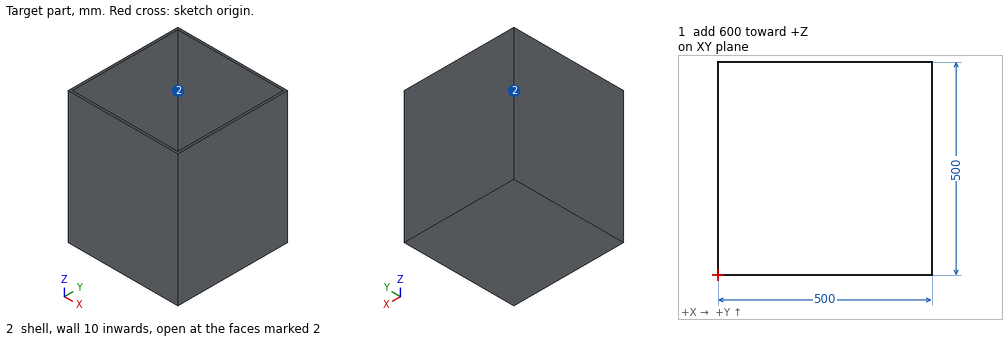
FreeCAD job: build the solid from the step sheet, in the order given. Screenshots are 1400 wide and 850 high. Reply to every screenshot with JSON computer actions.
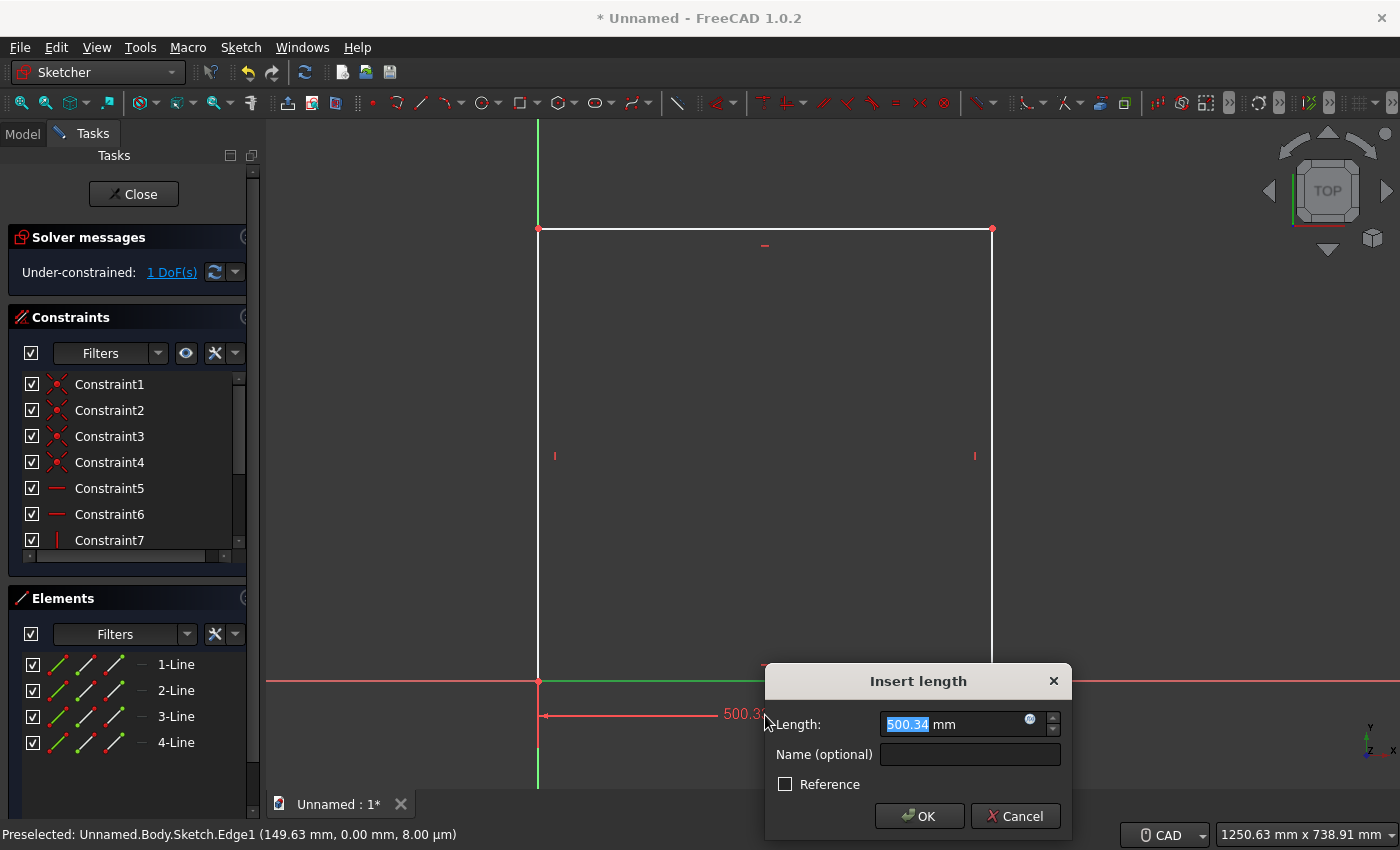
{"action": "type", "text": "500"}
{"action": "key", "text": "Return"}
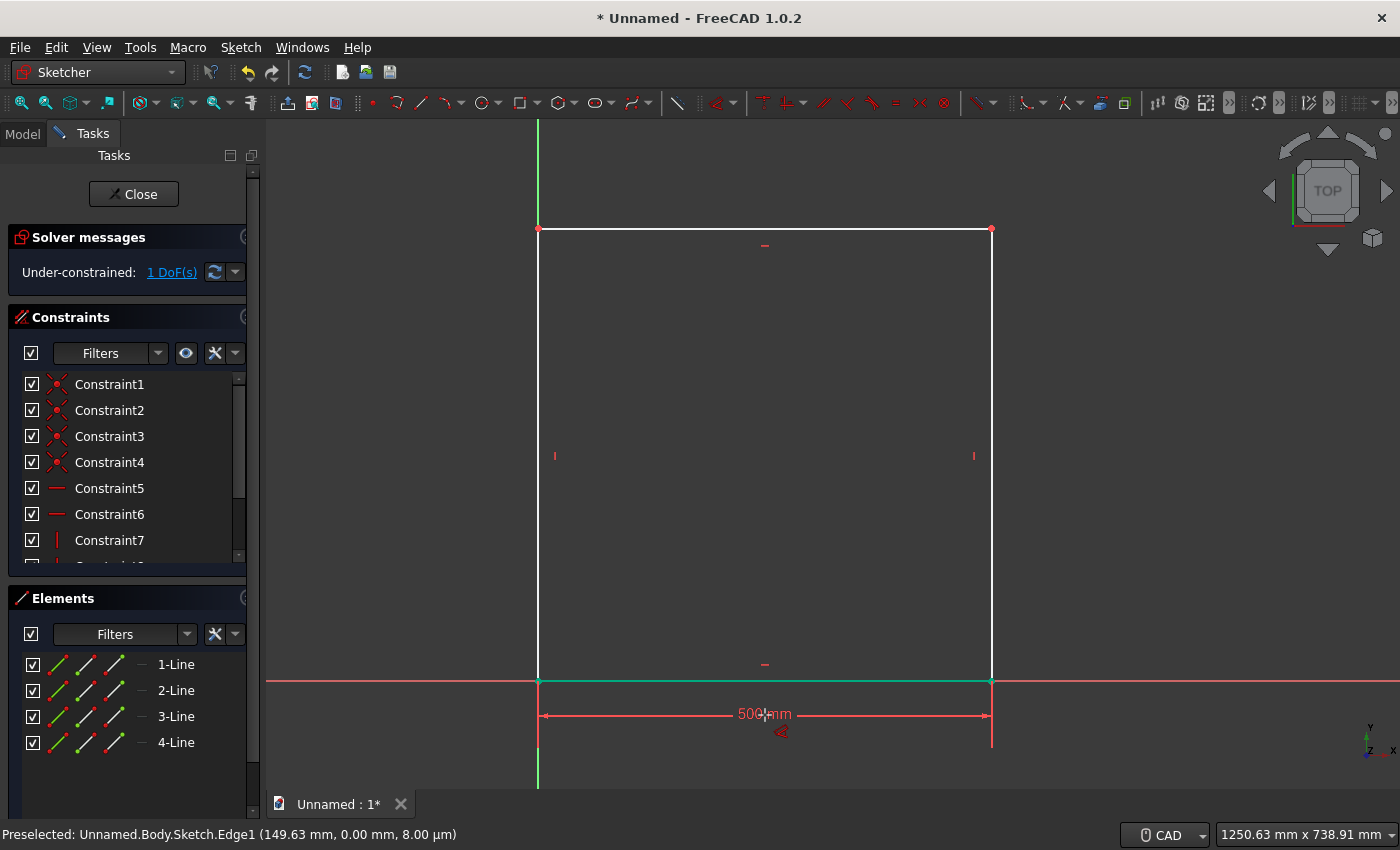
{"action": "left_click", "coordinate": [992, 546]}
{"action": "left_click", "coordinate": [1026, 455]}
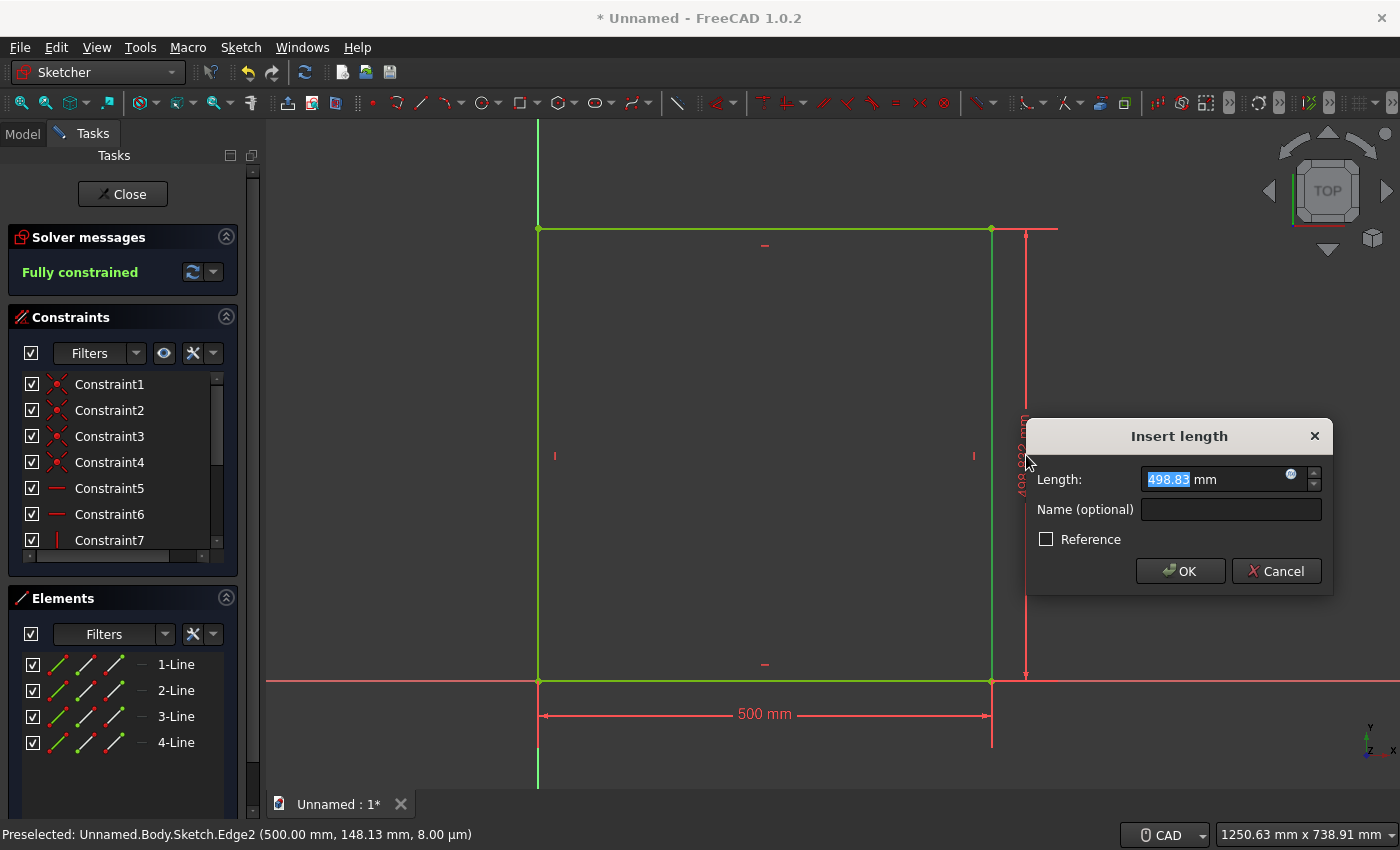
{"action": "type", "text": "500"}
{"action": "key", "text": "Return"}
{"action": "key", "text": "Escape"}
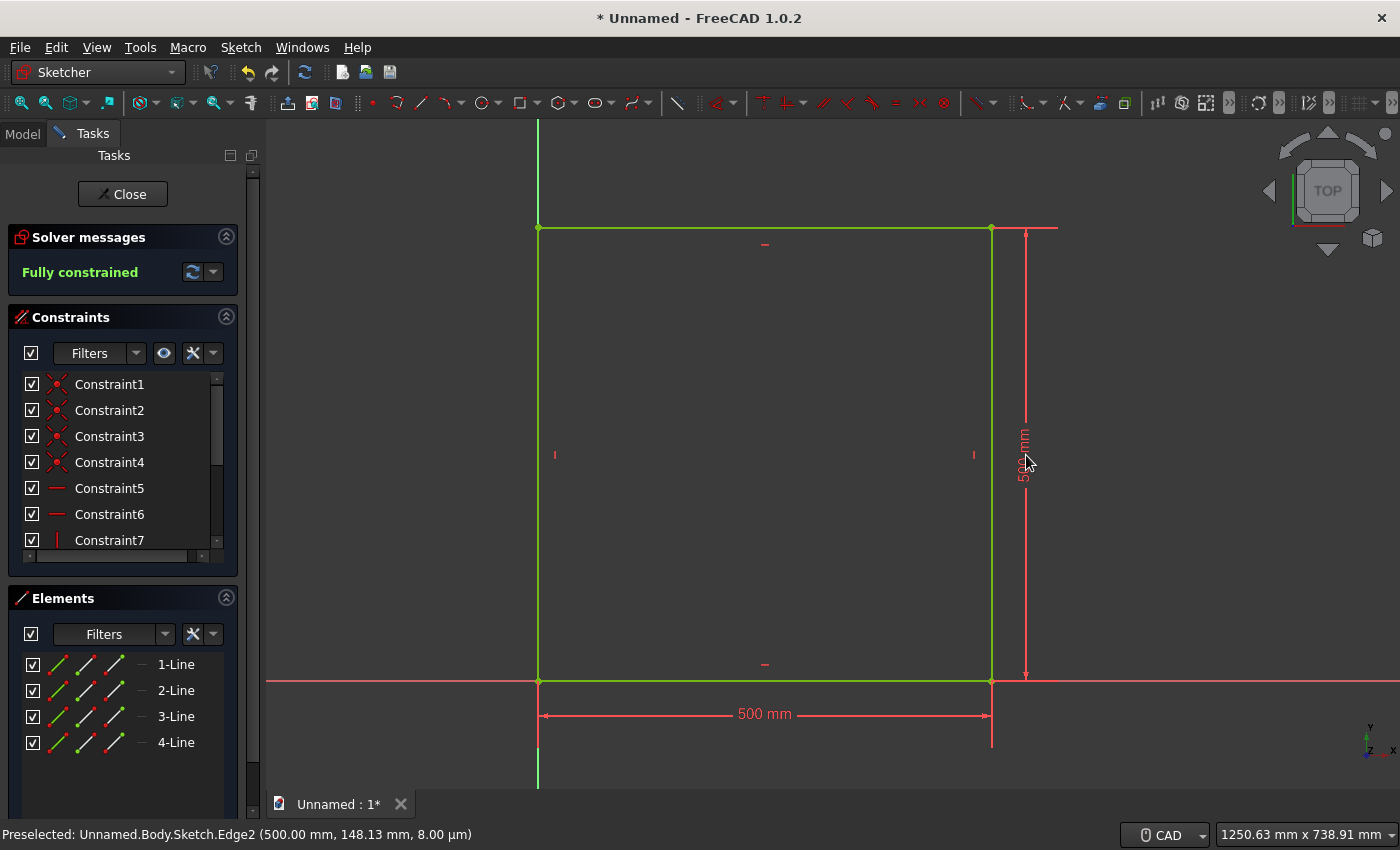
{"action": "left_click", "coordinate": [123, 194]}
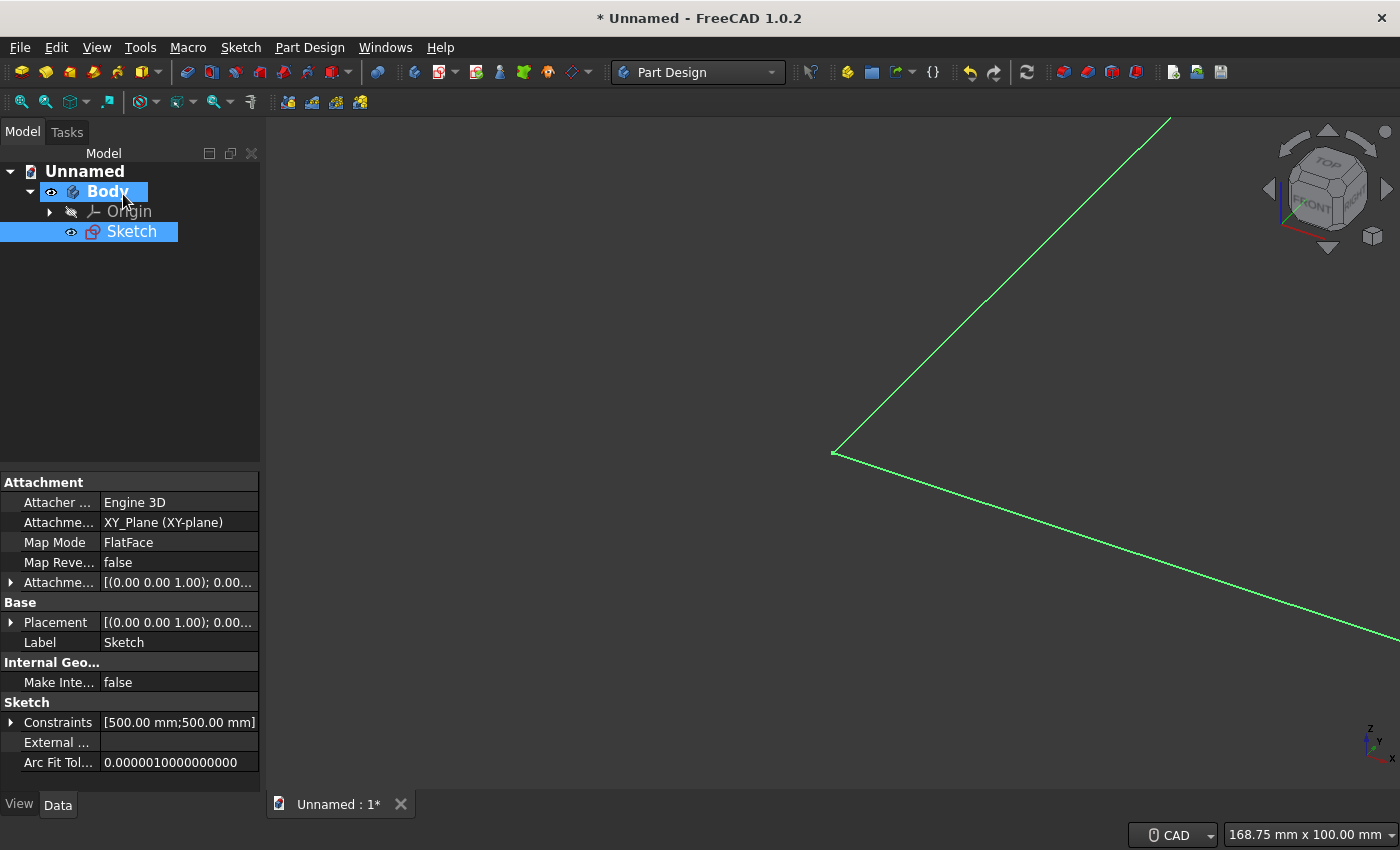
{"action": "left_click", "coordinate": [22, 72]}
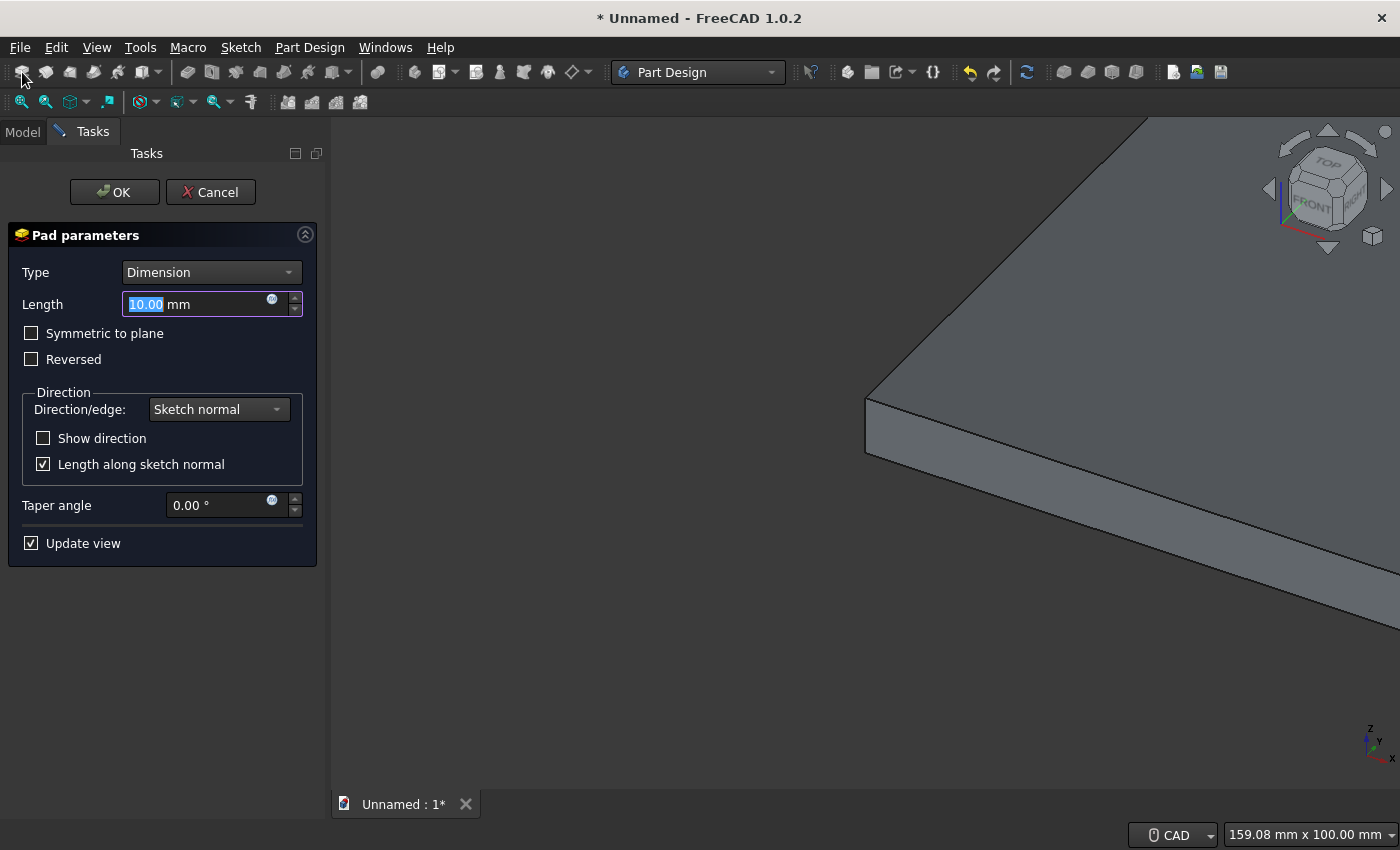
{"action": "type", "text": "600"}
{"action": "key", "text": "Tab"}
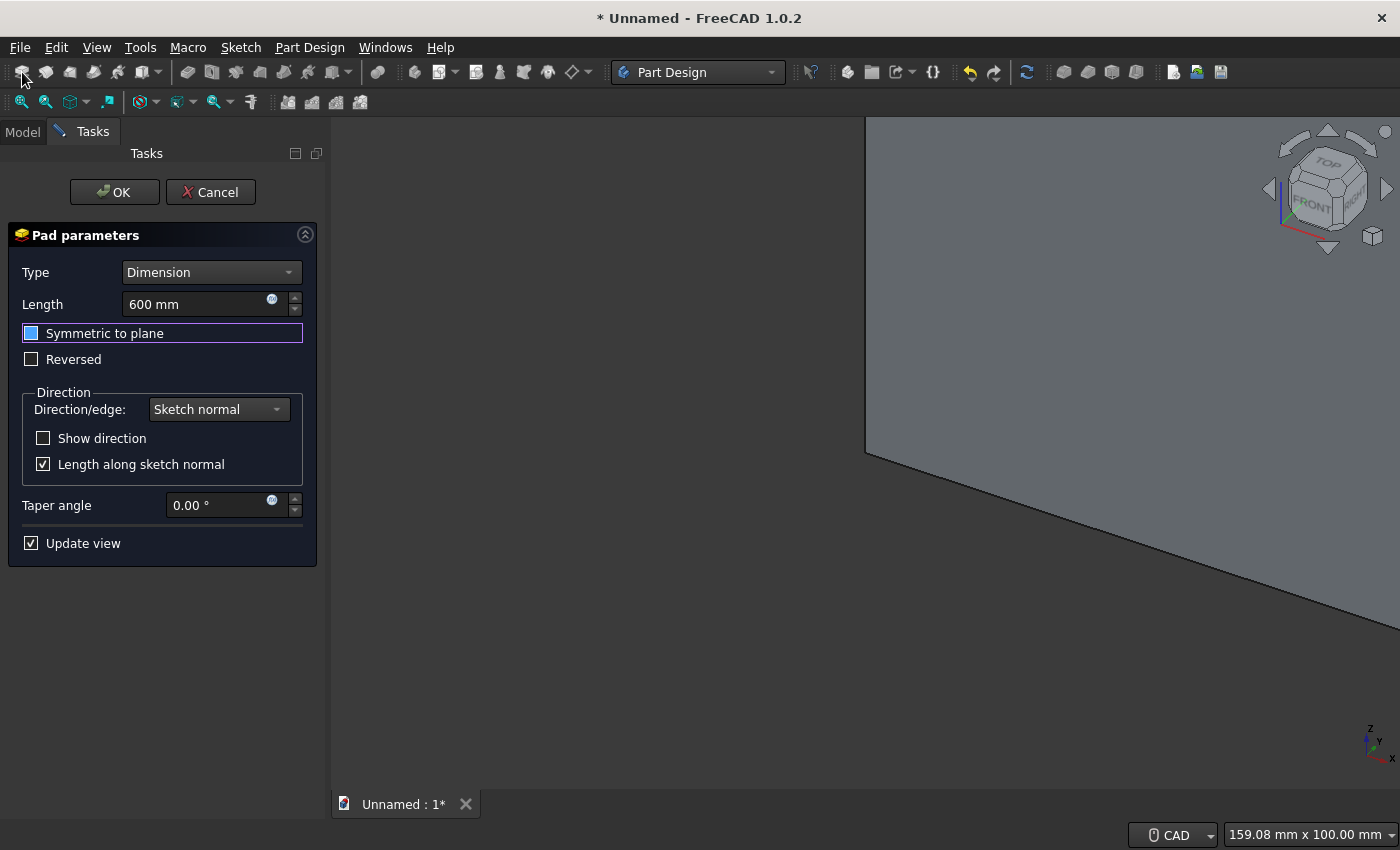
{"action": "left_click", "coordinate": [115, 192]}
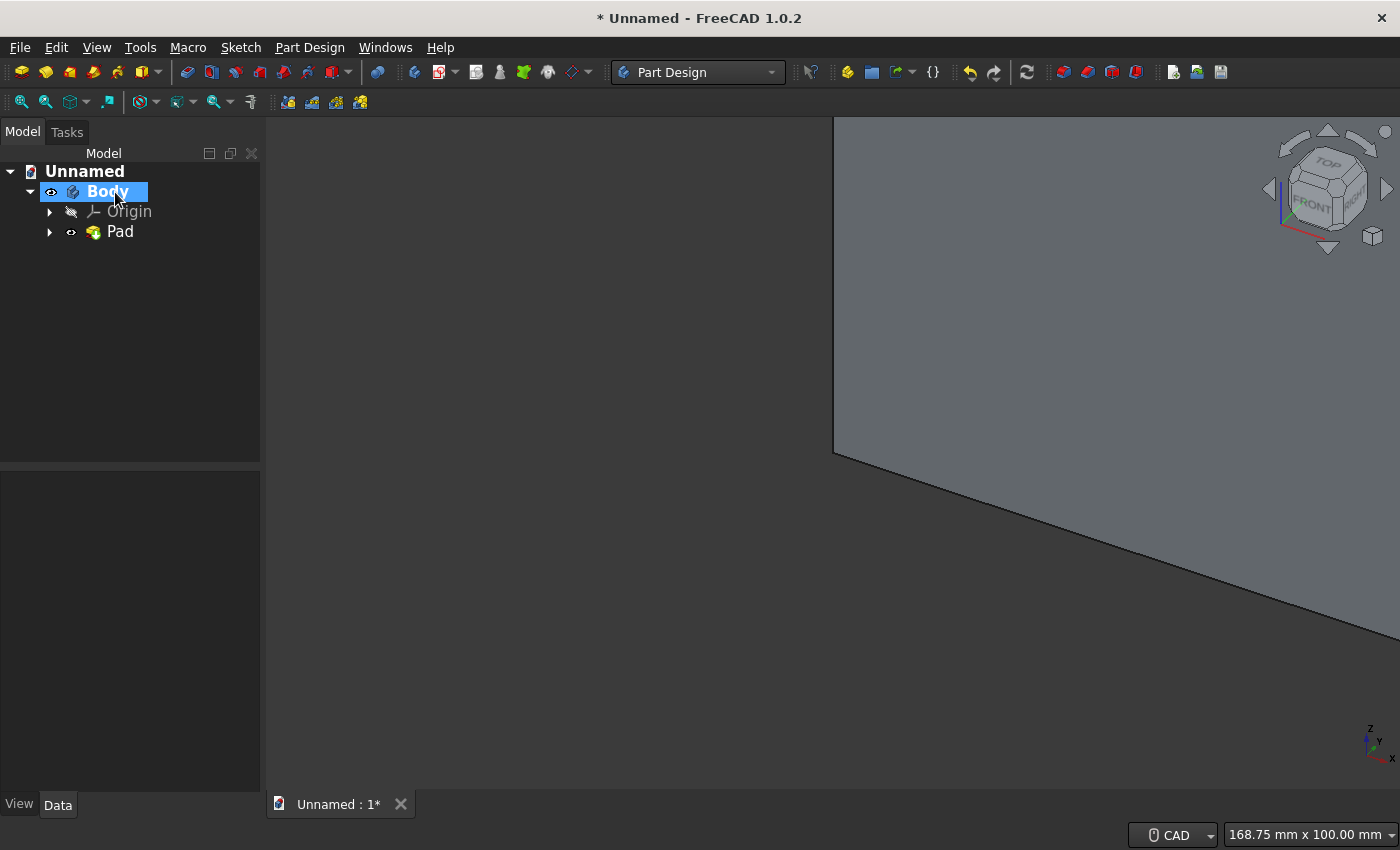
{"action": "left_click", "coordinate": [22, 102]}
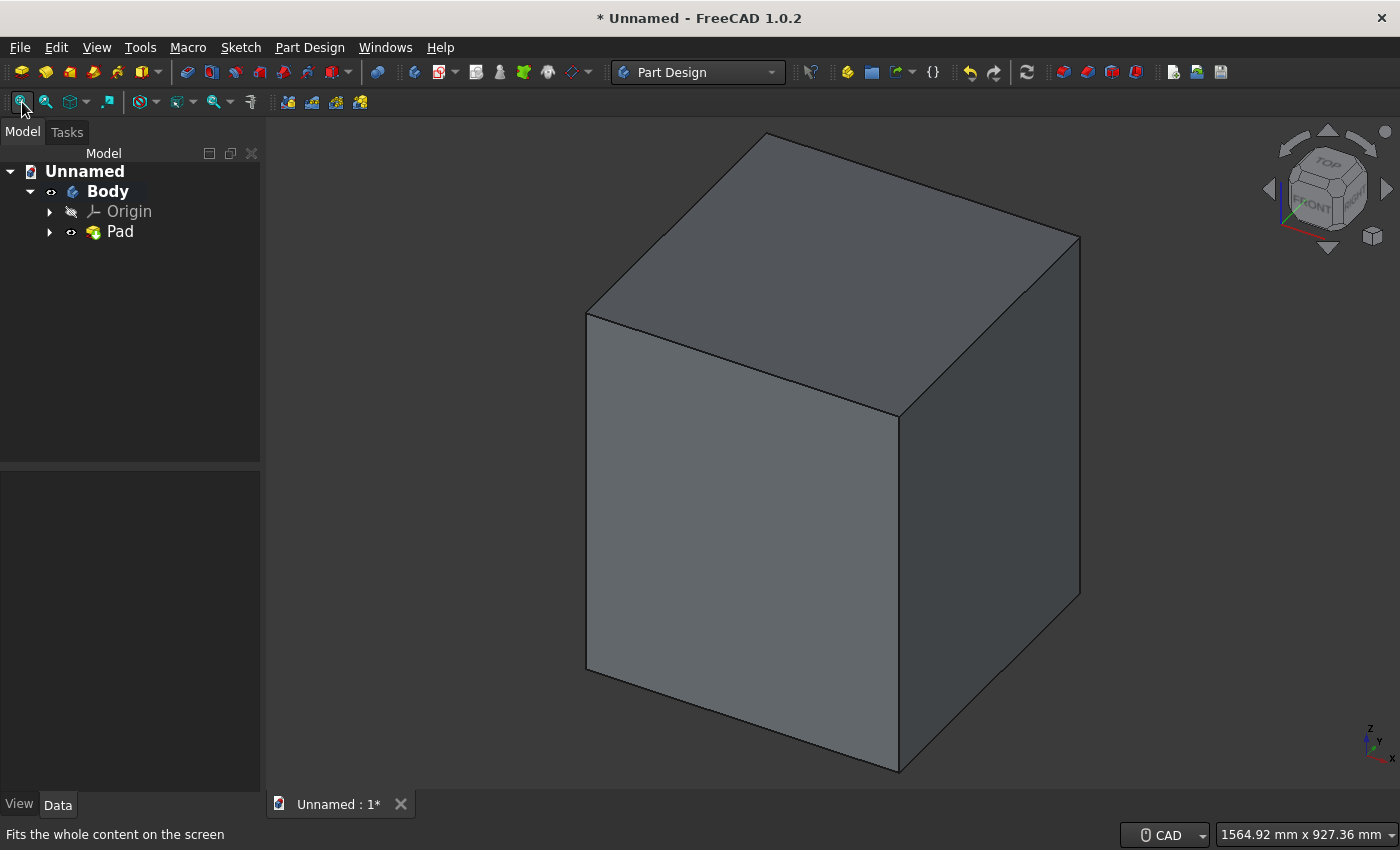
{"action": "left_click", "coordinate": [833, 274]}